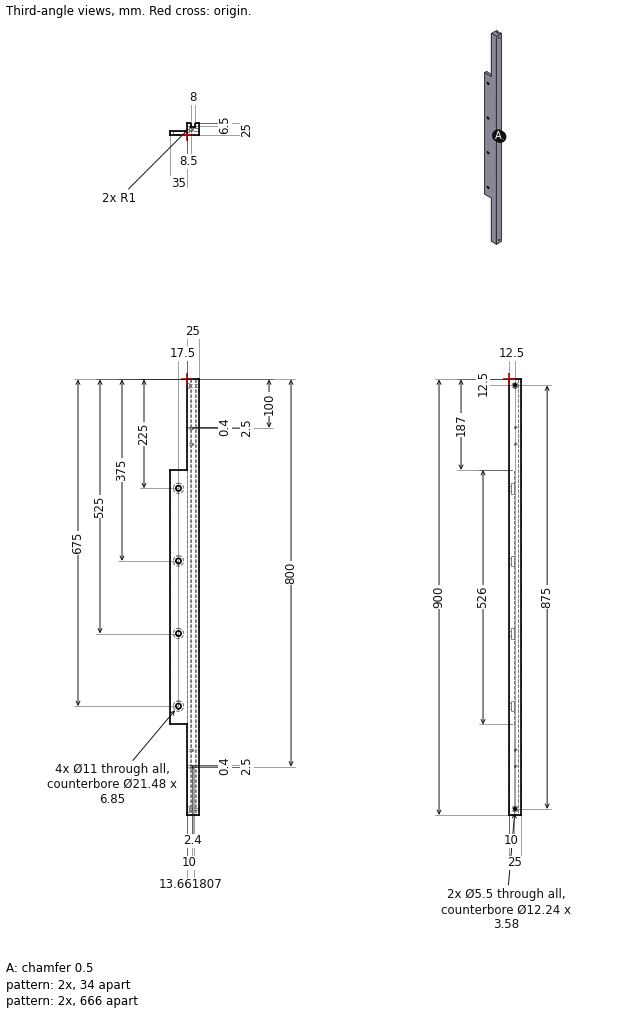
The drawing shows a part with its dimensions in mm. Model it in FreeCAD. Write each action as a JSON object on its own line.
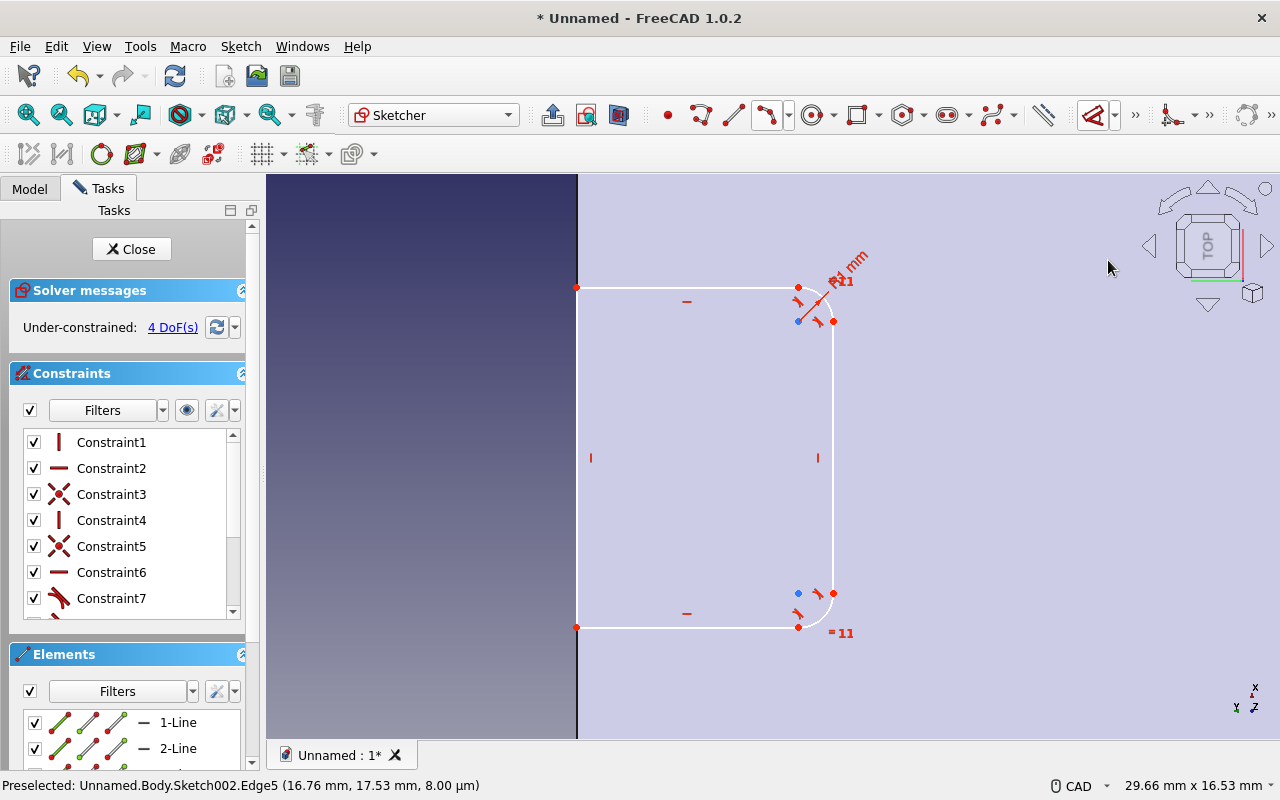
{"action": "left_click", "coordinate": [833, 512]}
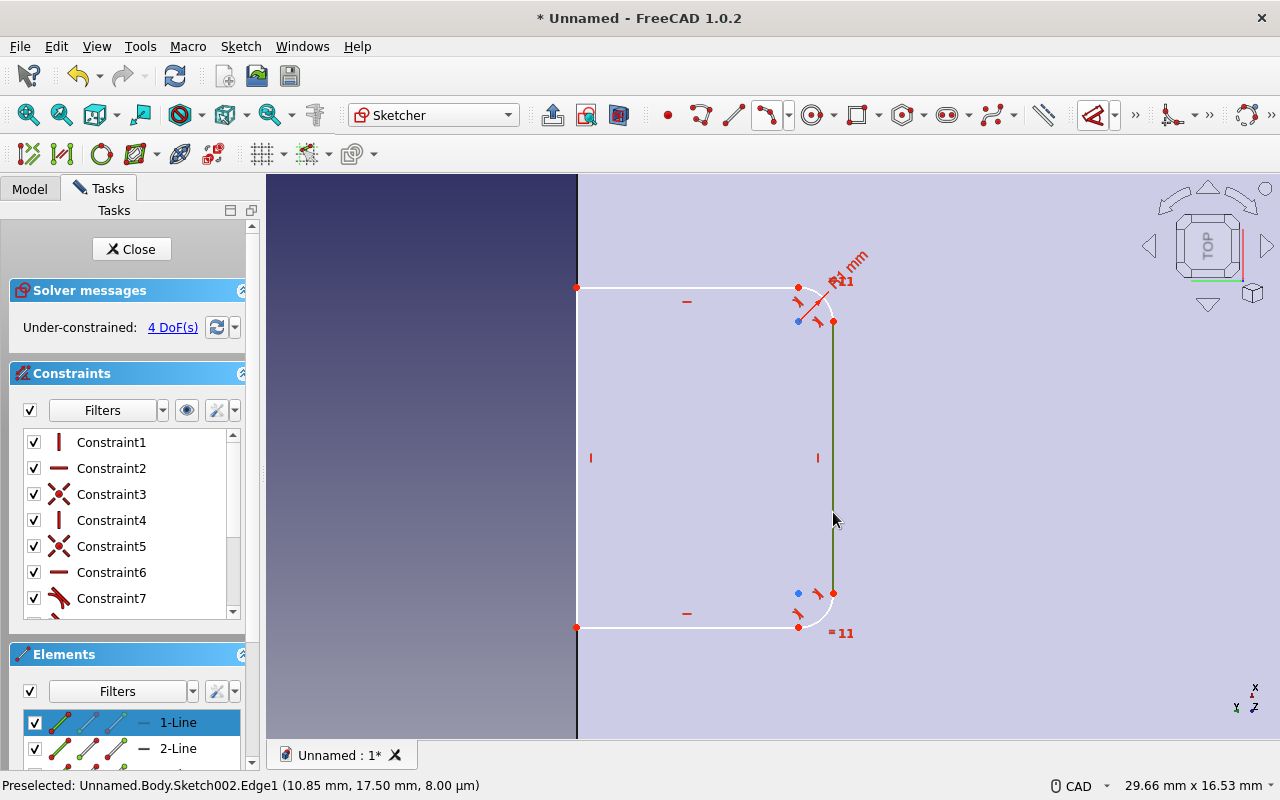
{"action": "key", "text": "i"}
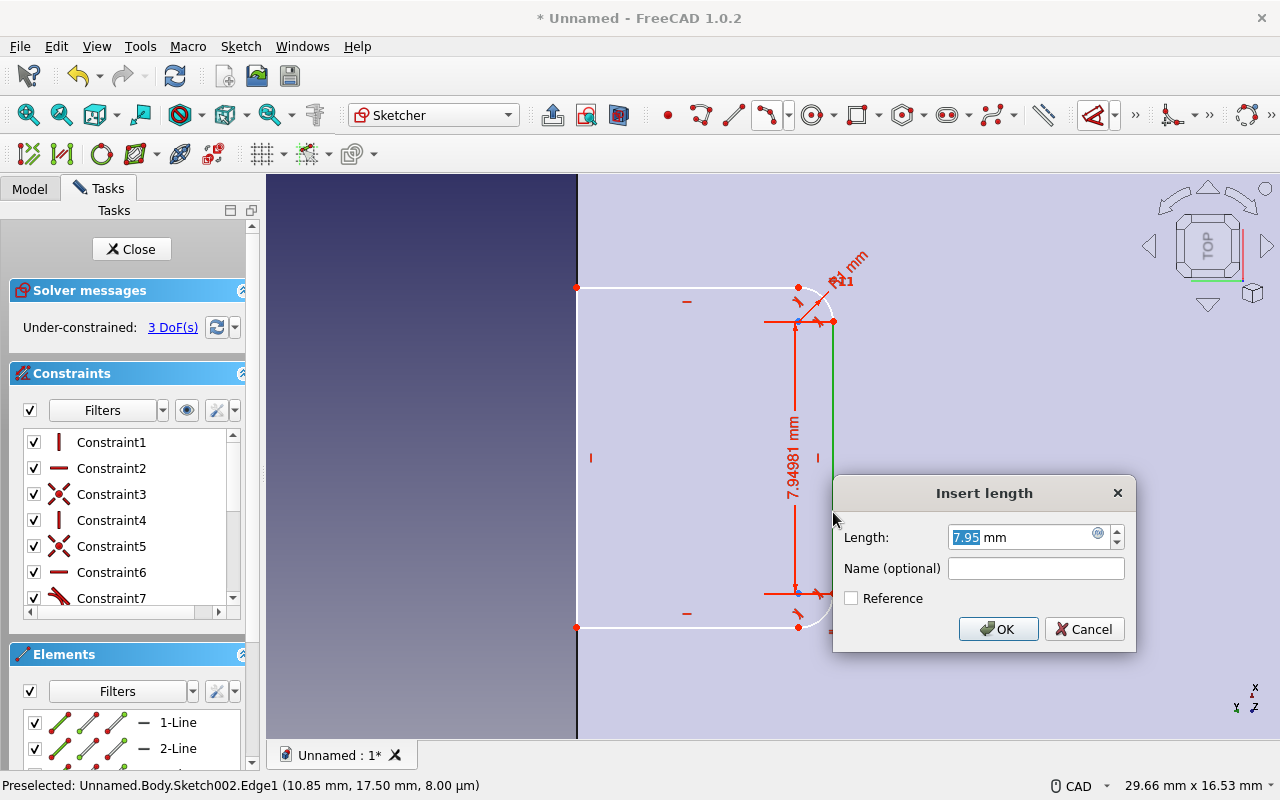
{"action": "type", "text": "8"}
{"action": "key", "text": "Return"}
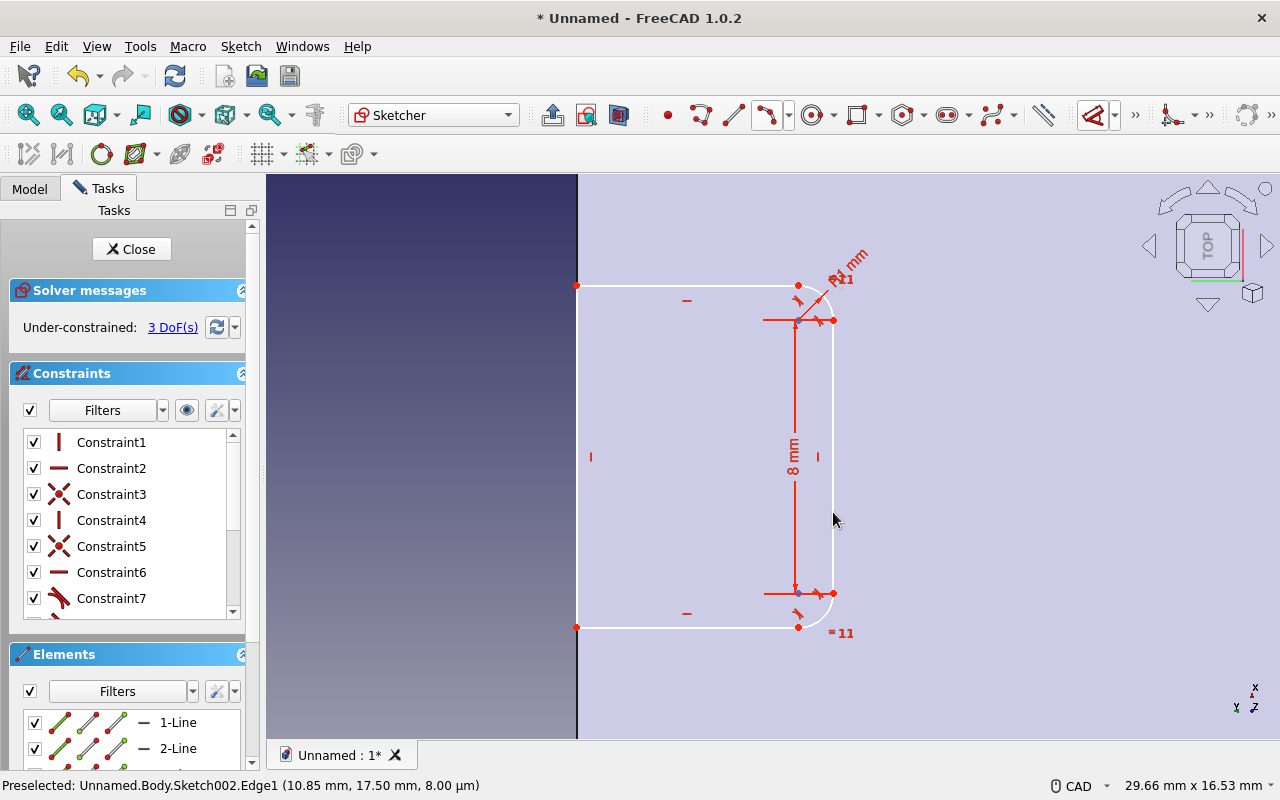
{"action": "left_click", "coordinate": [732, 286]}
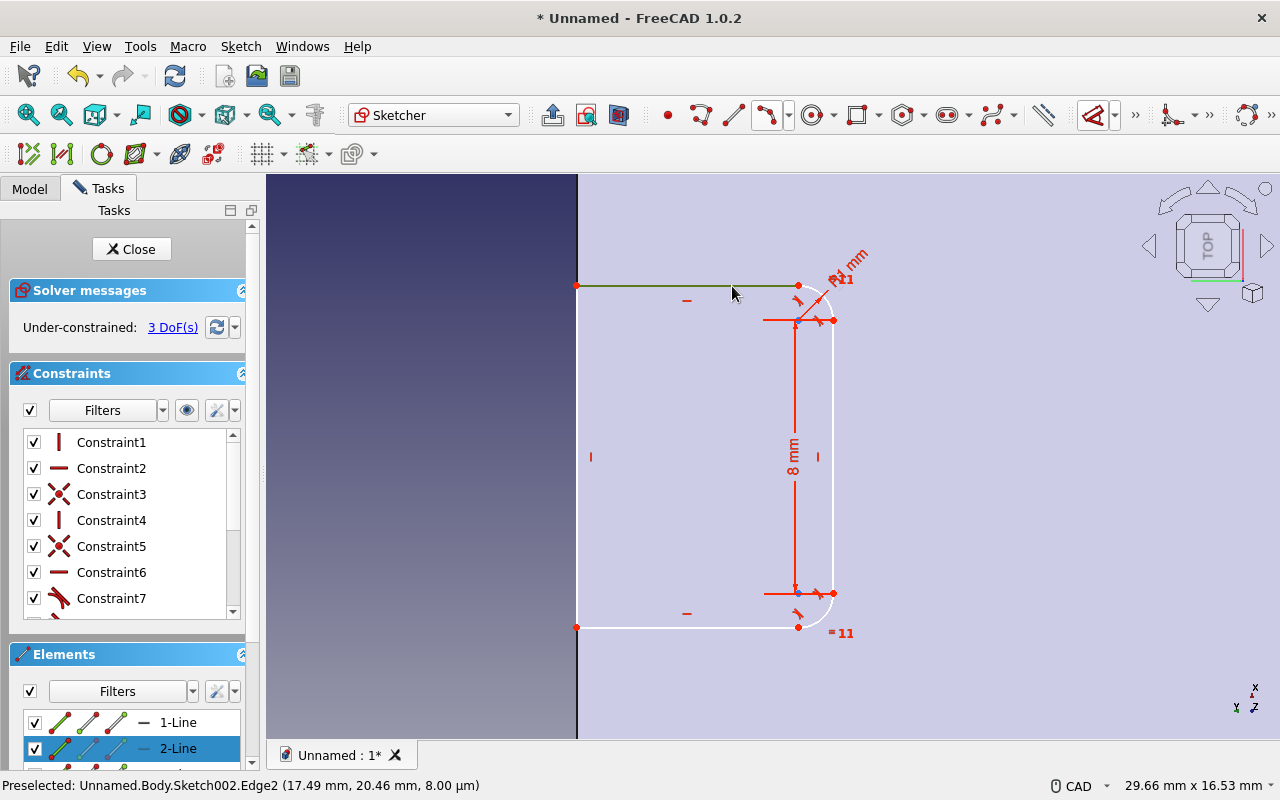
{"action": "left_click", "coordinate": [1114, 116]}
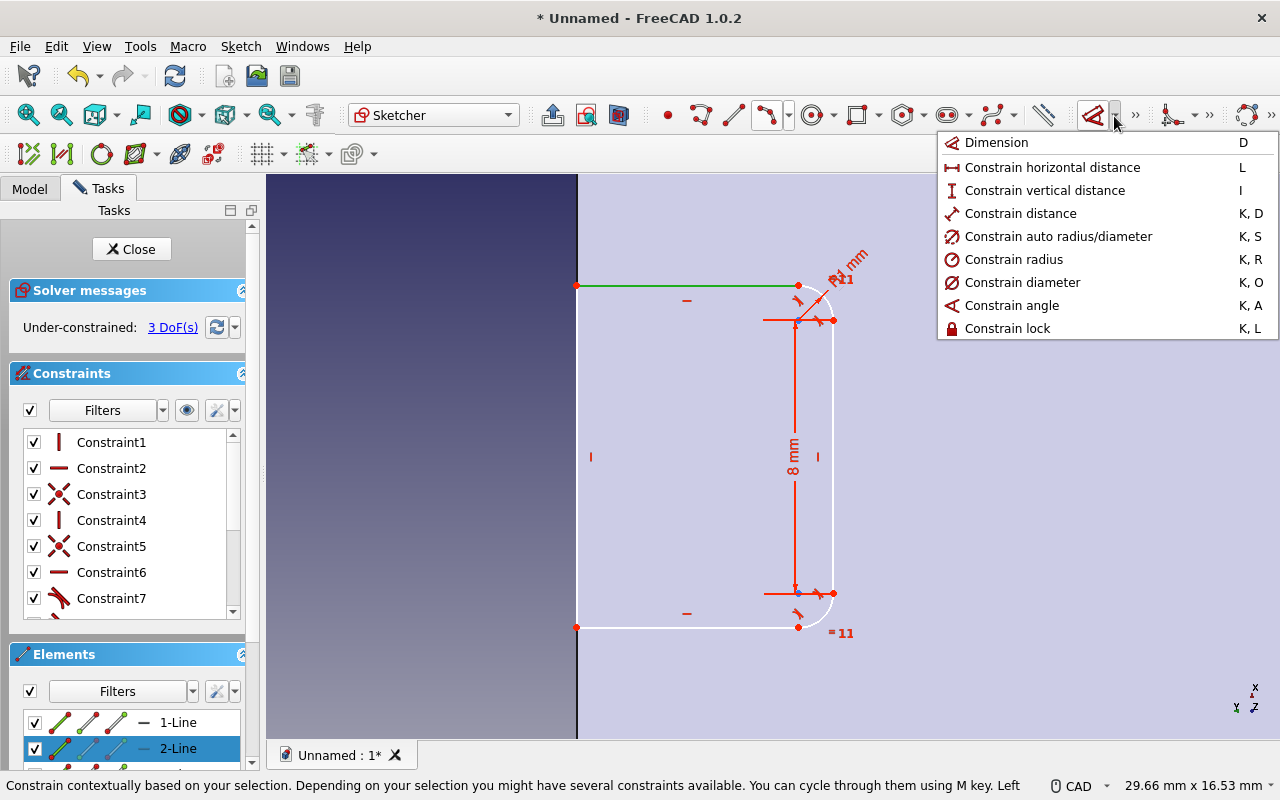
{"action": "left_click", "coordinate": [1108, 168]}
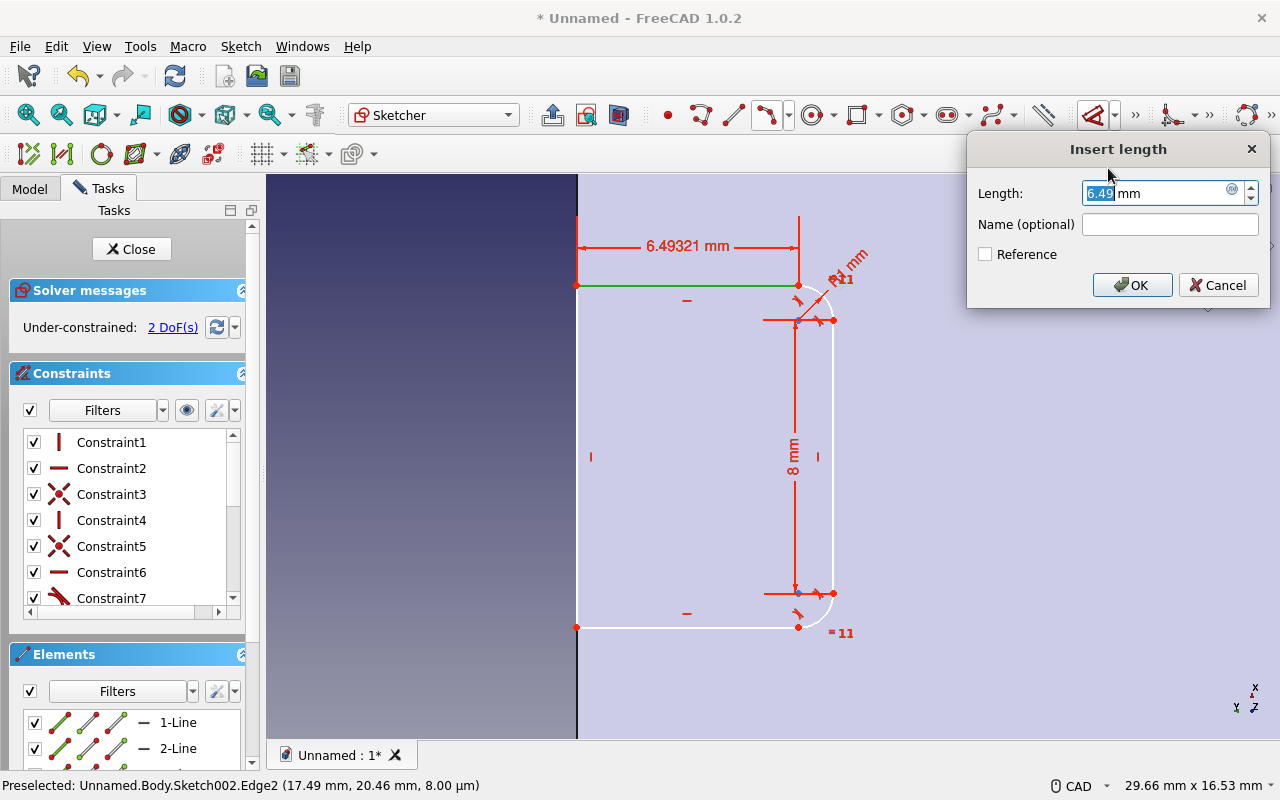
{"action": "type", "text": "6.5"}
{"action": "key", "text": "Return"}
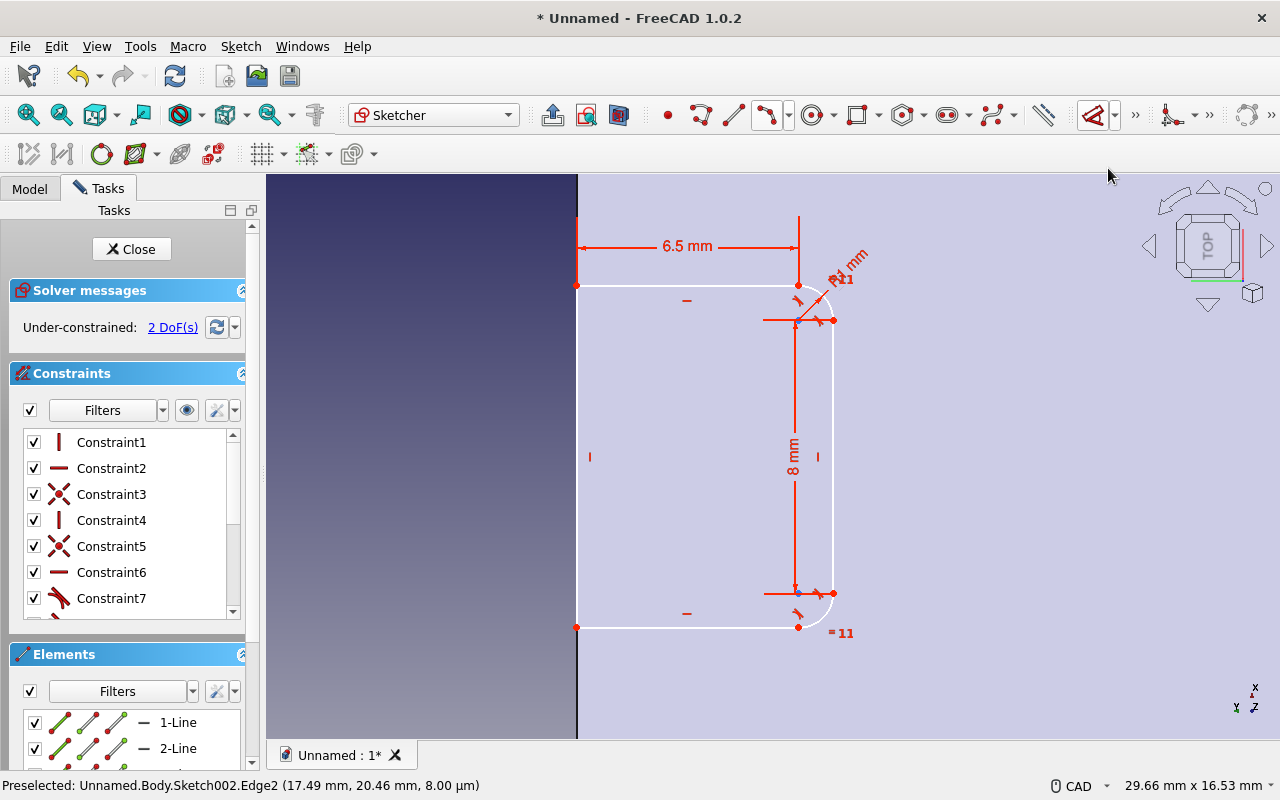
{"action": "left_click", "coordinate": [577, 286]}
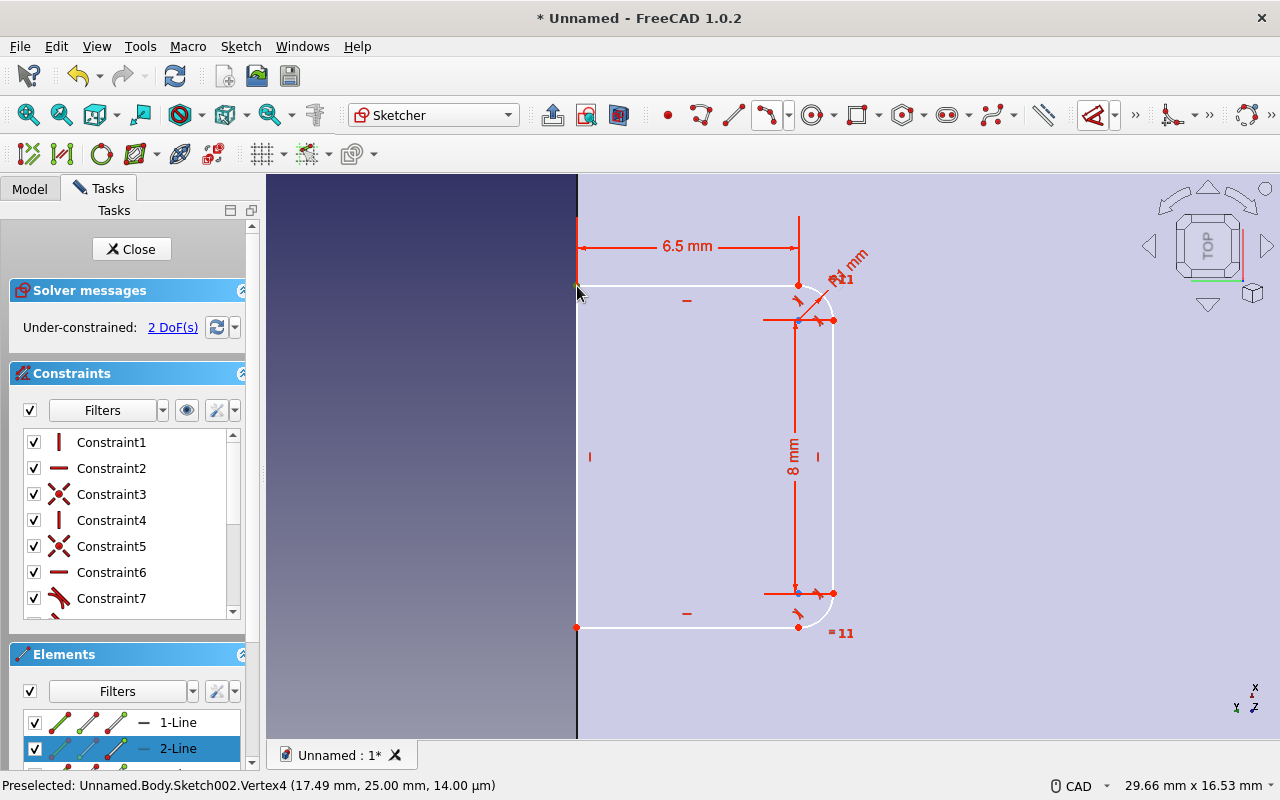
{"action": "key", "text": "l"}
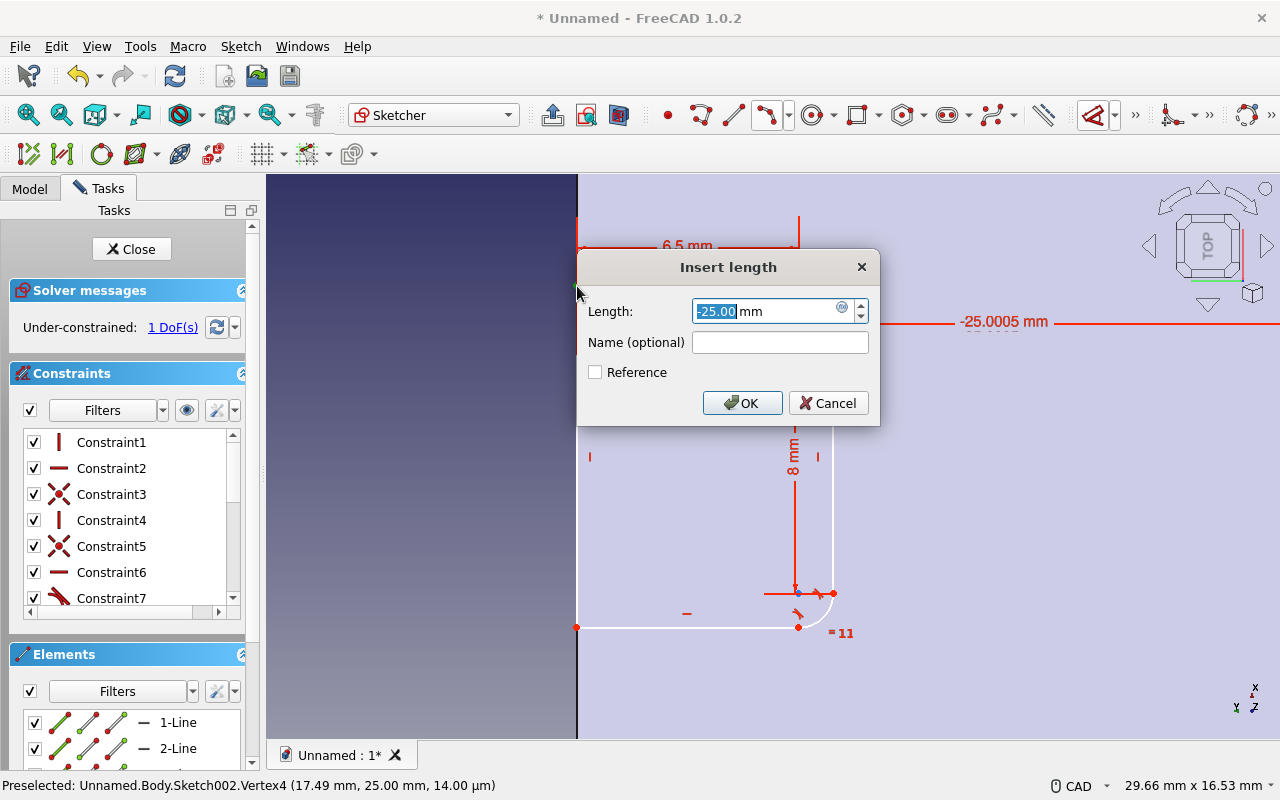
{"action": "type", "text": "-25"}
{"action": "key", "text": "Return"}